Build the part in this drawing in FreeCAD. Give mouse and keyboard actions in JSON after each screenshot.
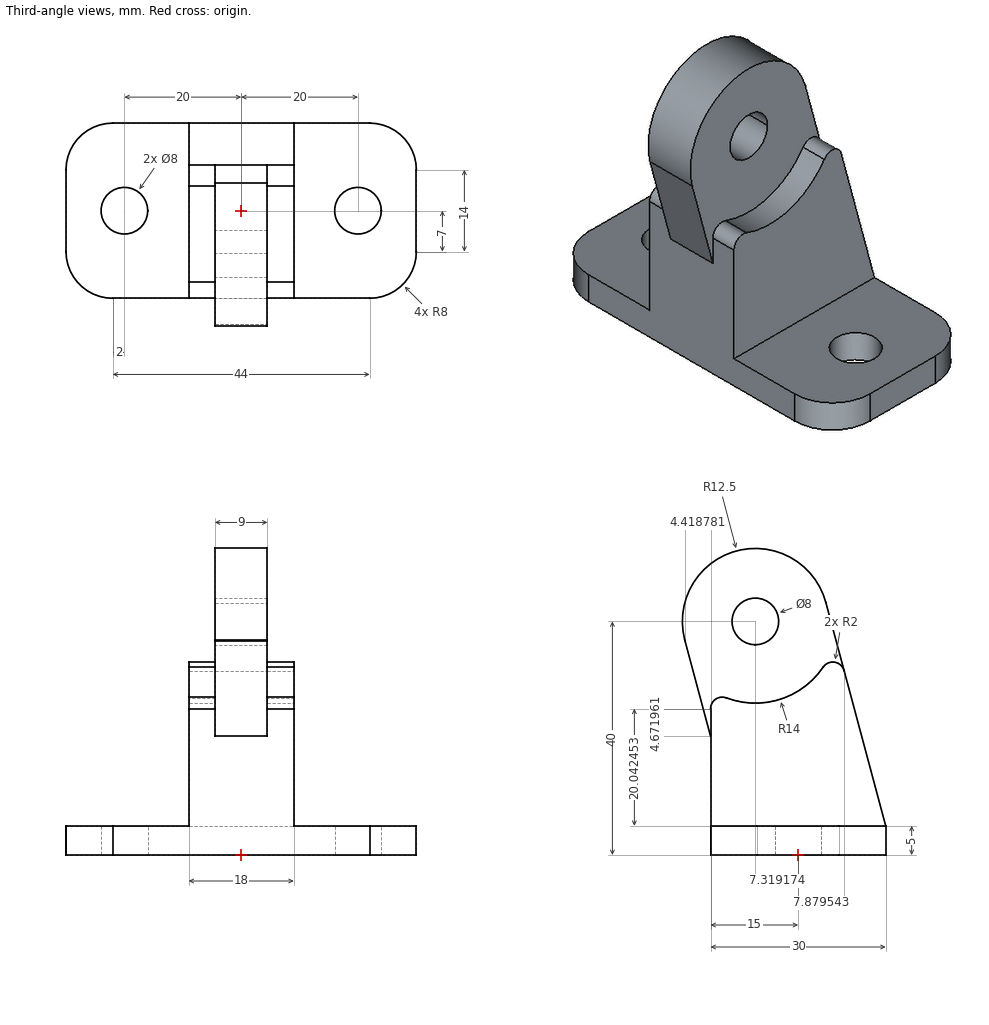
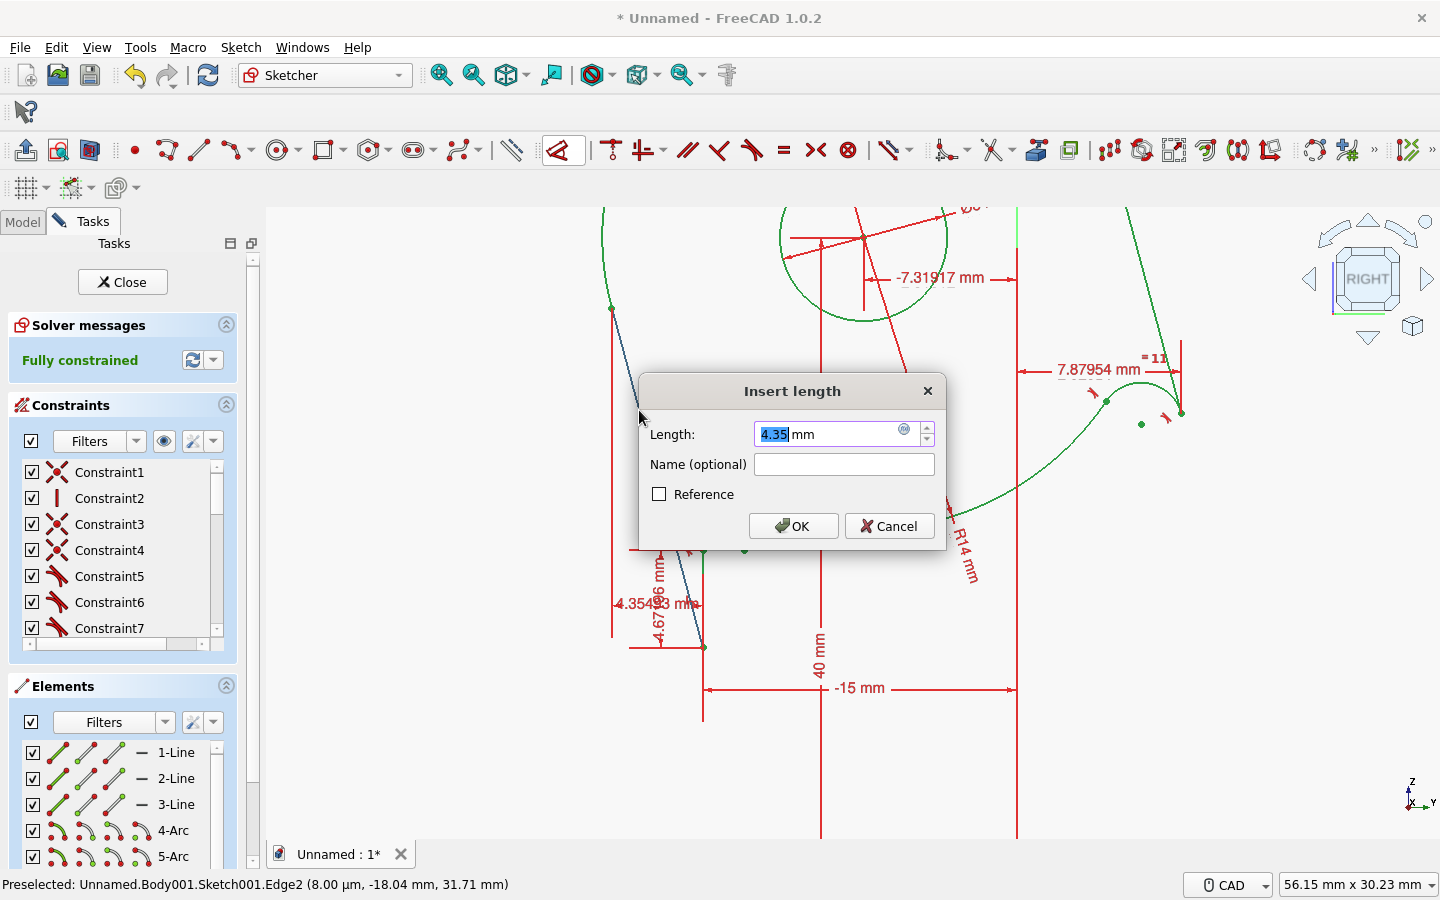
{"action": "type", "text": "4.418781"}
{"action": "key", "text": "Return"}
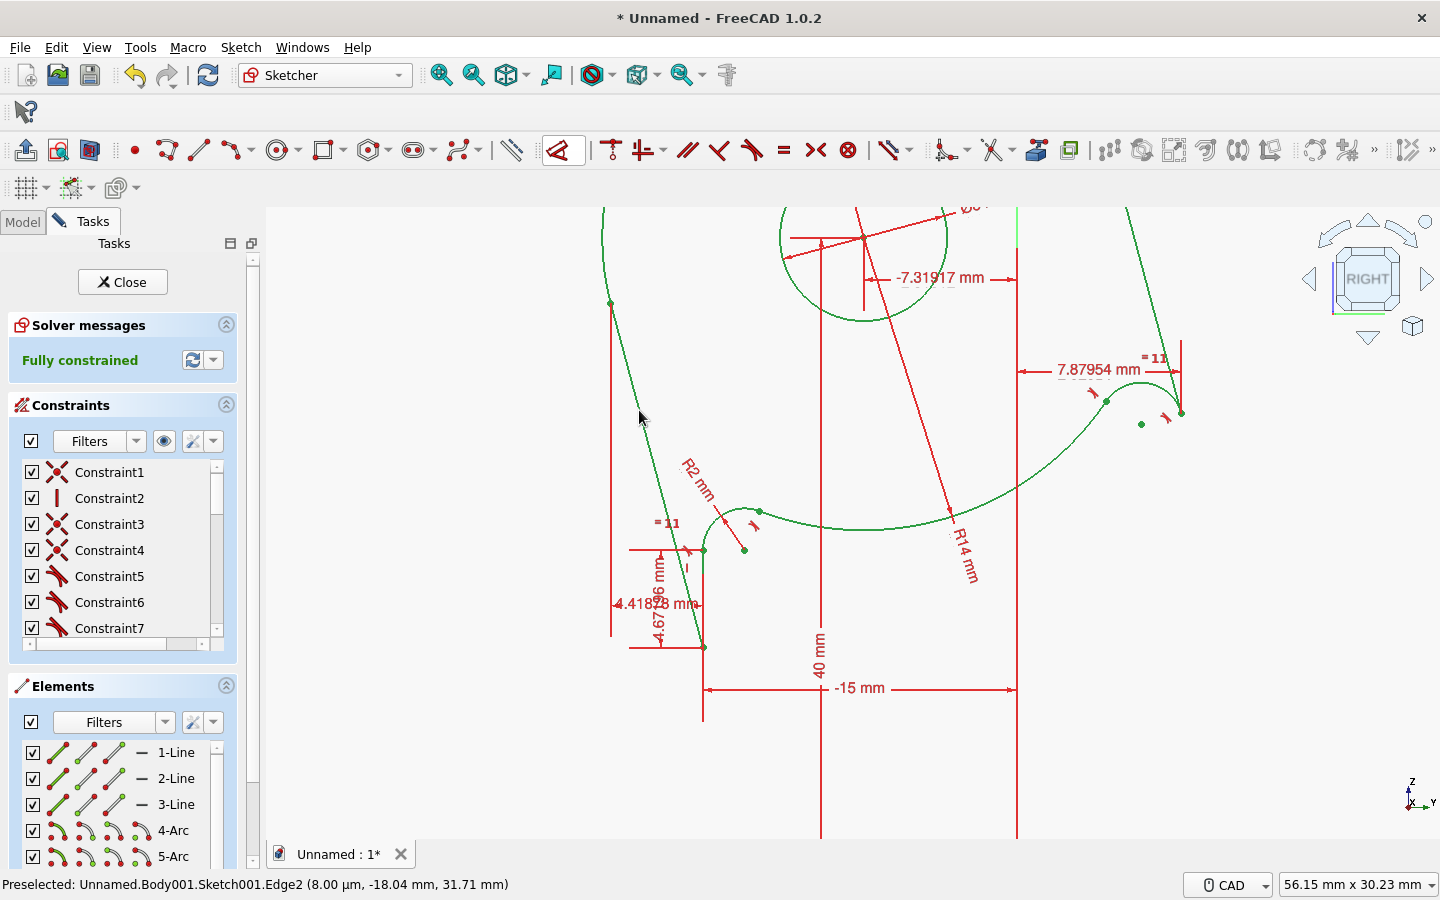
{"action": "left_click", "coordinate": [123, 282]}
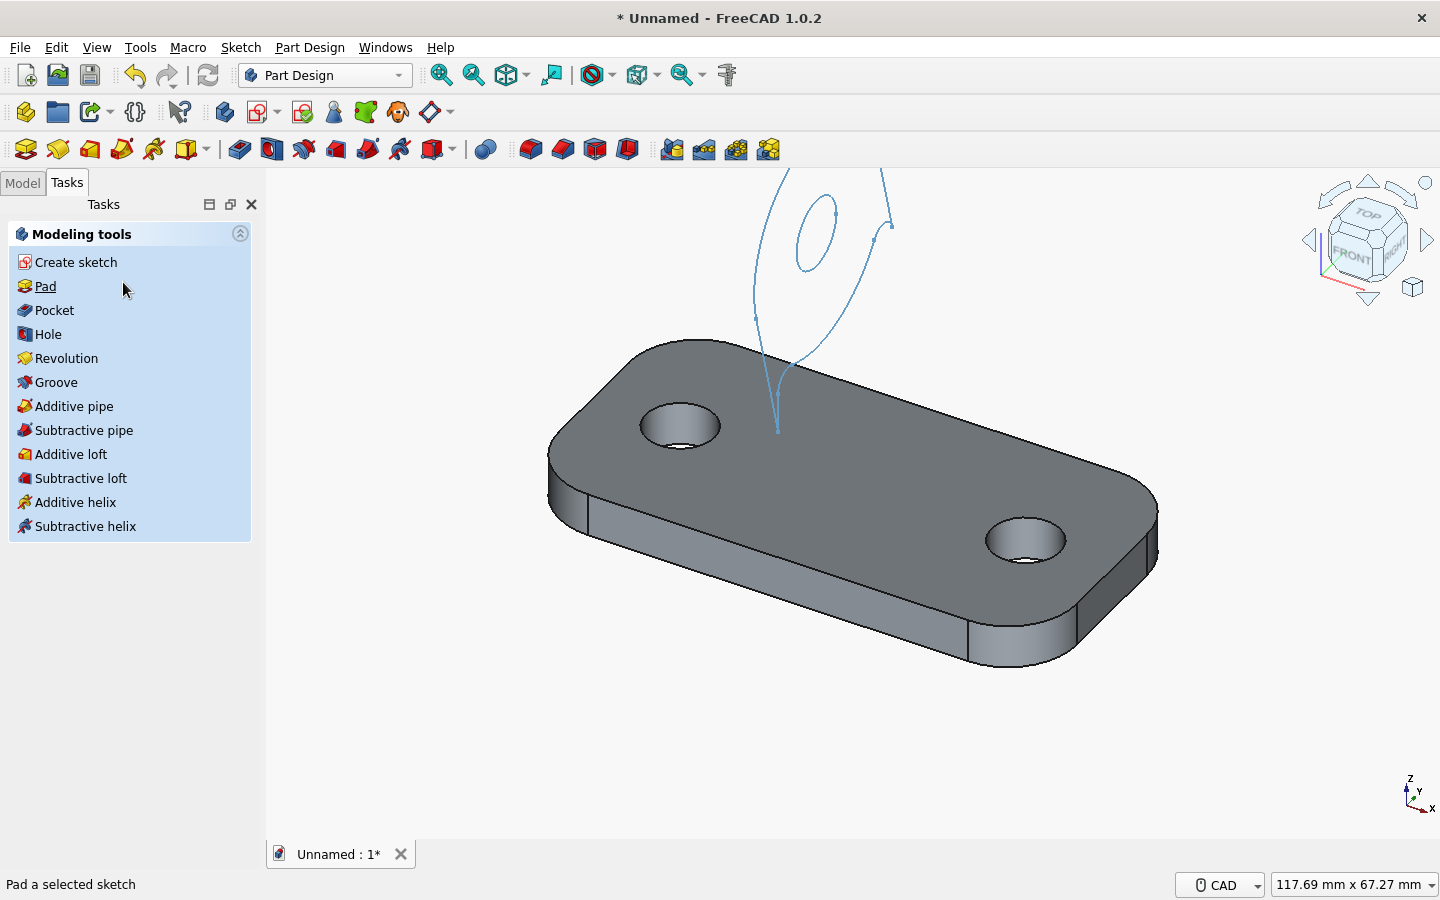
{"action": "left_click", "coordinate": [26, 150]}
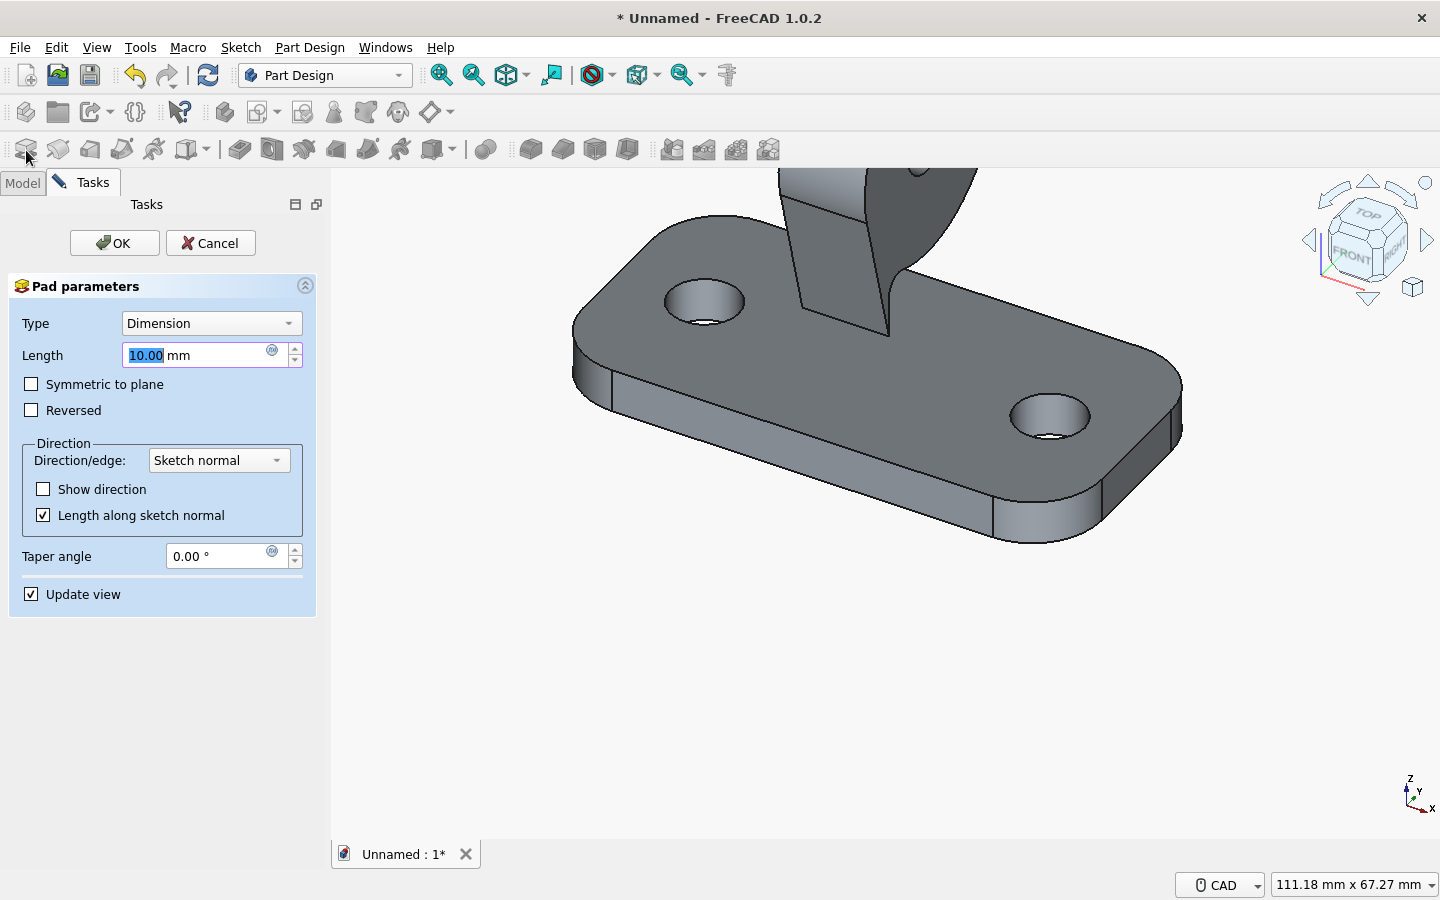
{"action": "type", "text": "9"}
{"action": "key", "text": "Tab"}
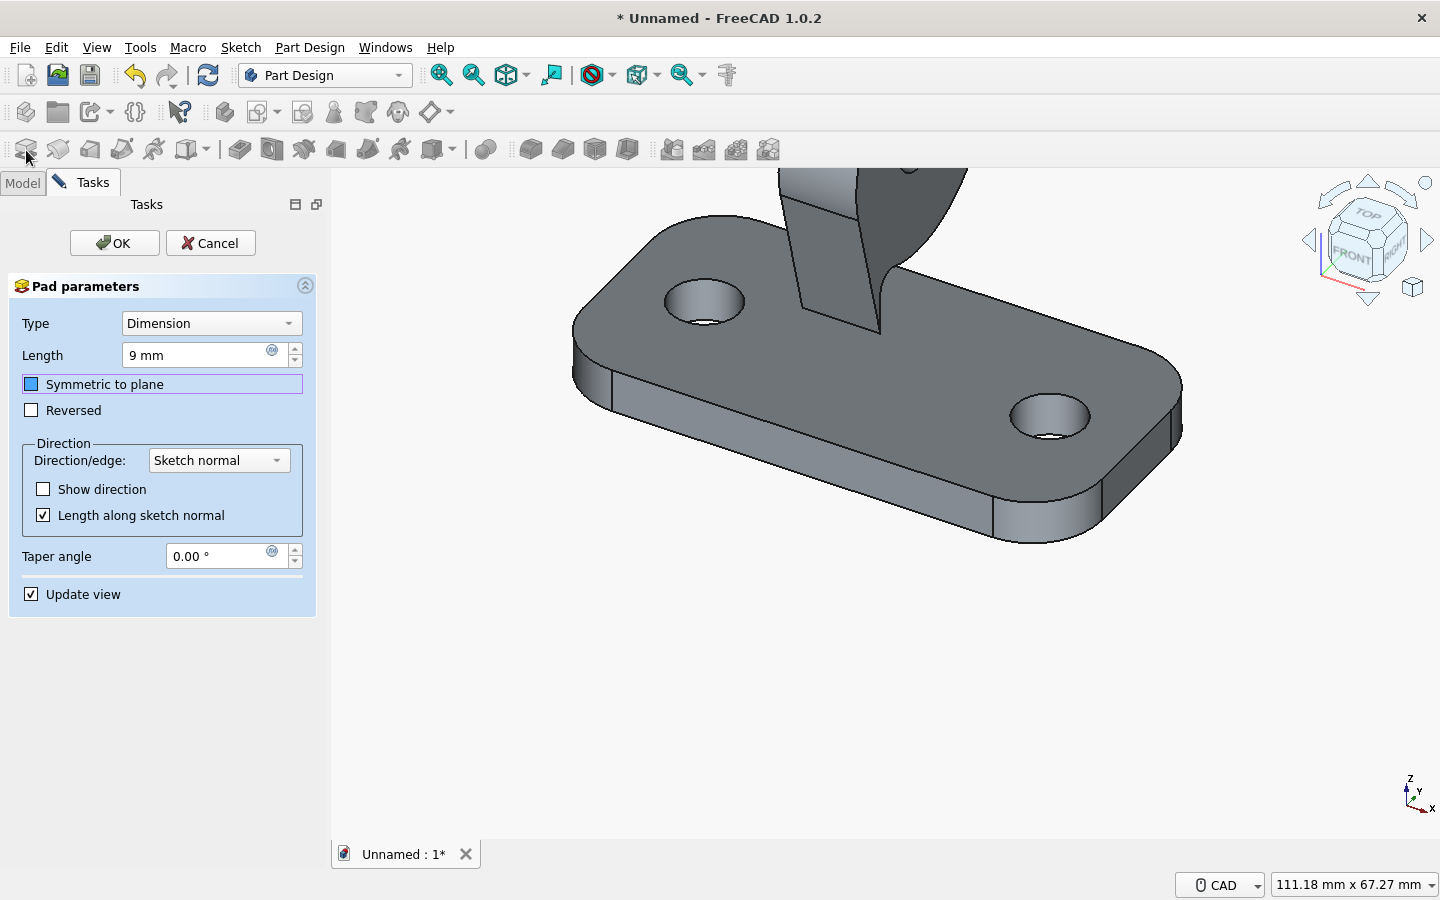
{"action": "left_click", "coordinate": [30, 384]}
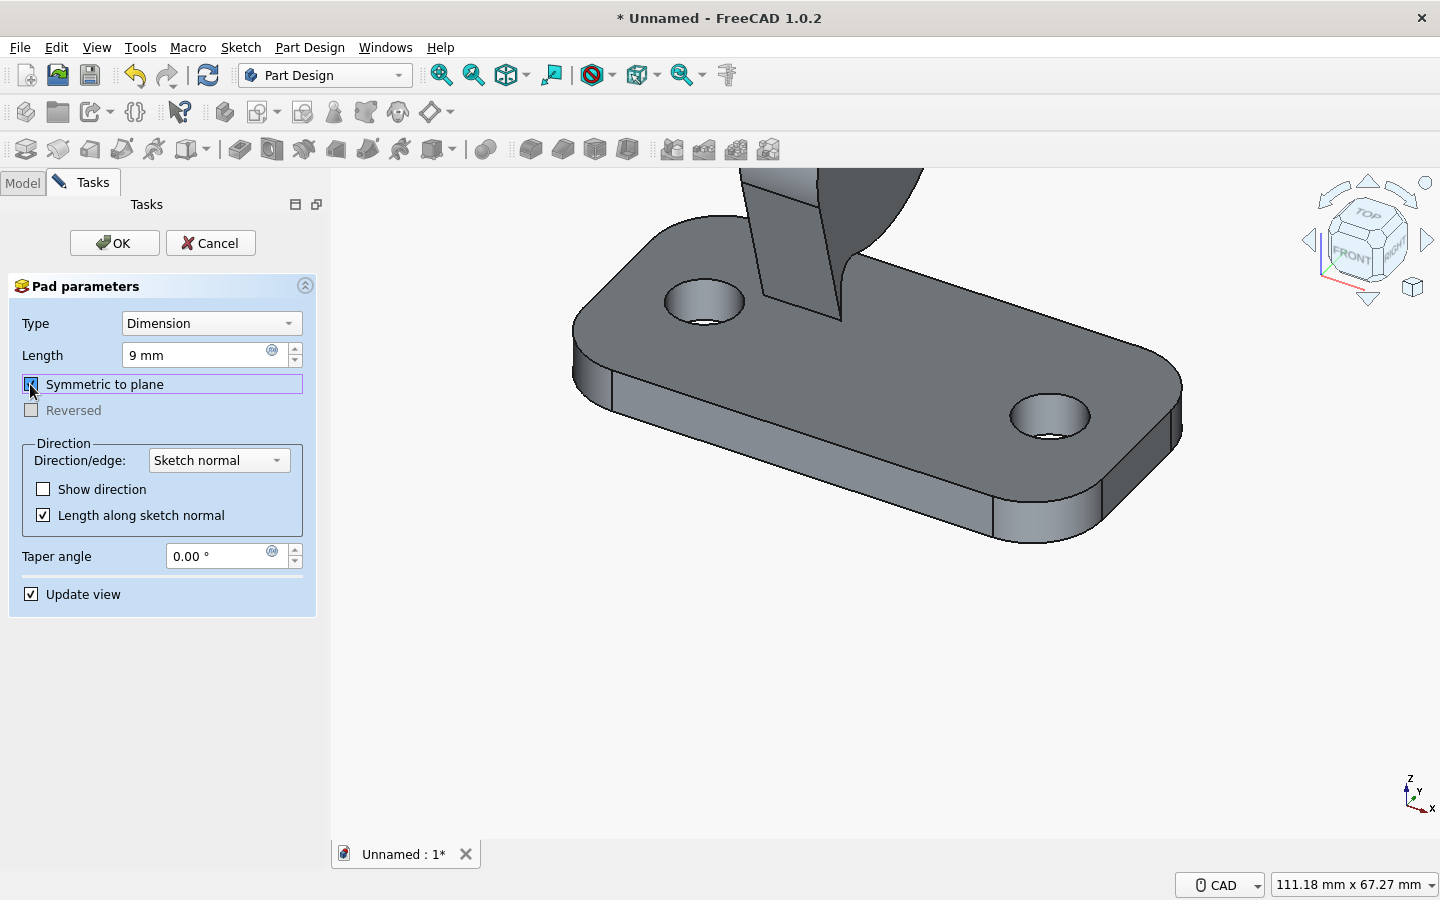
{"action": "left_click", "coordinate": [115, 243]}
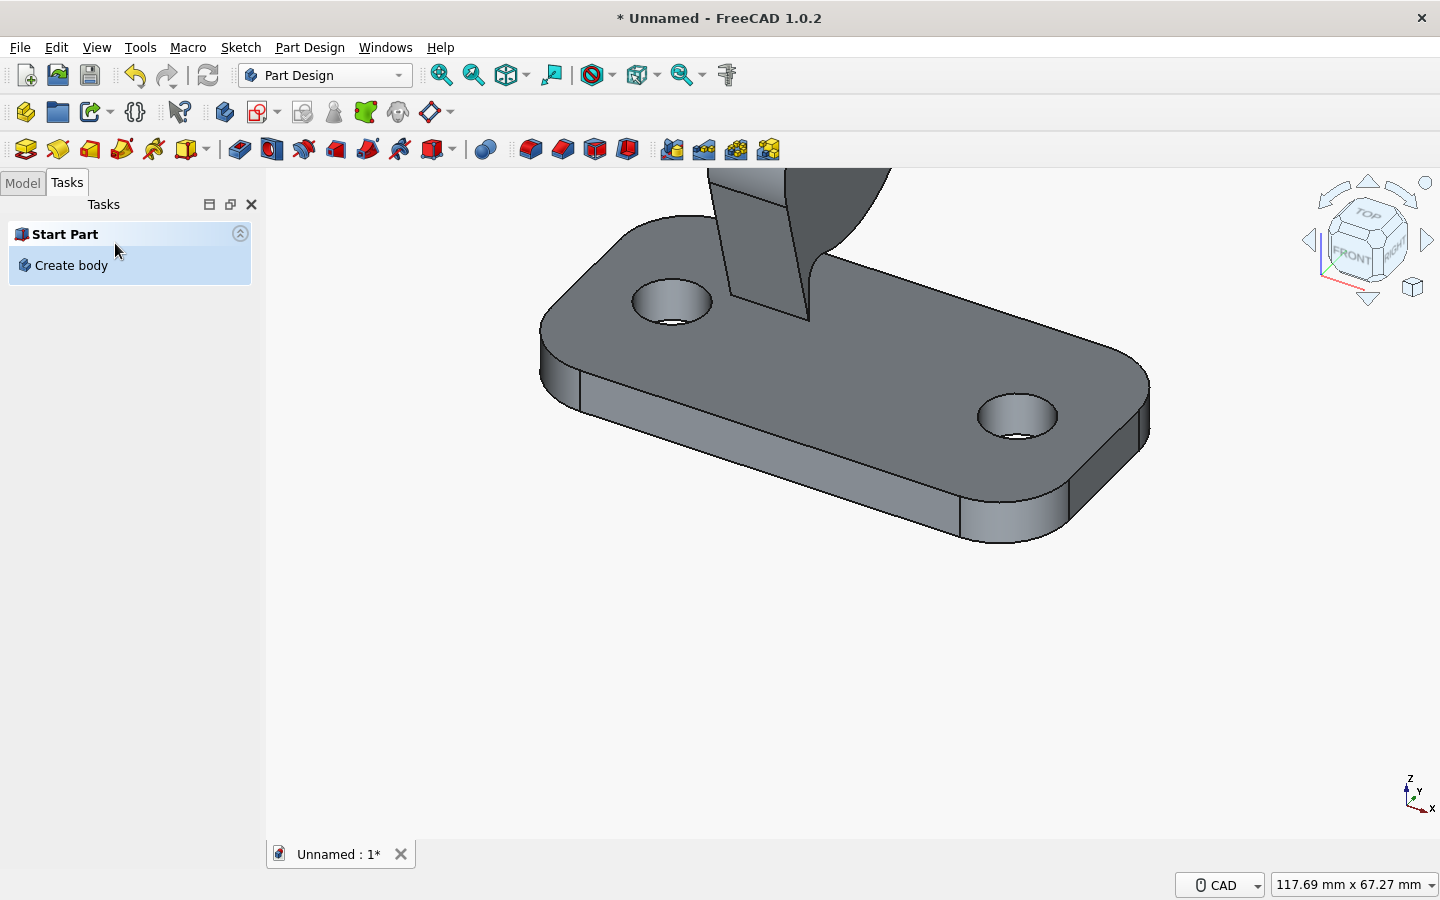
{"action": "left_click", "coordinate": [442, 76]}